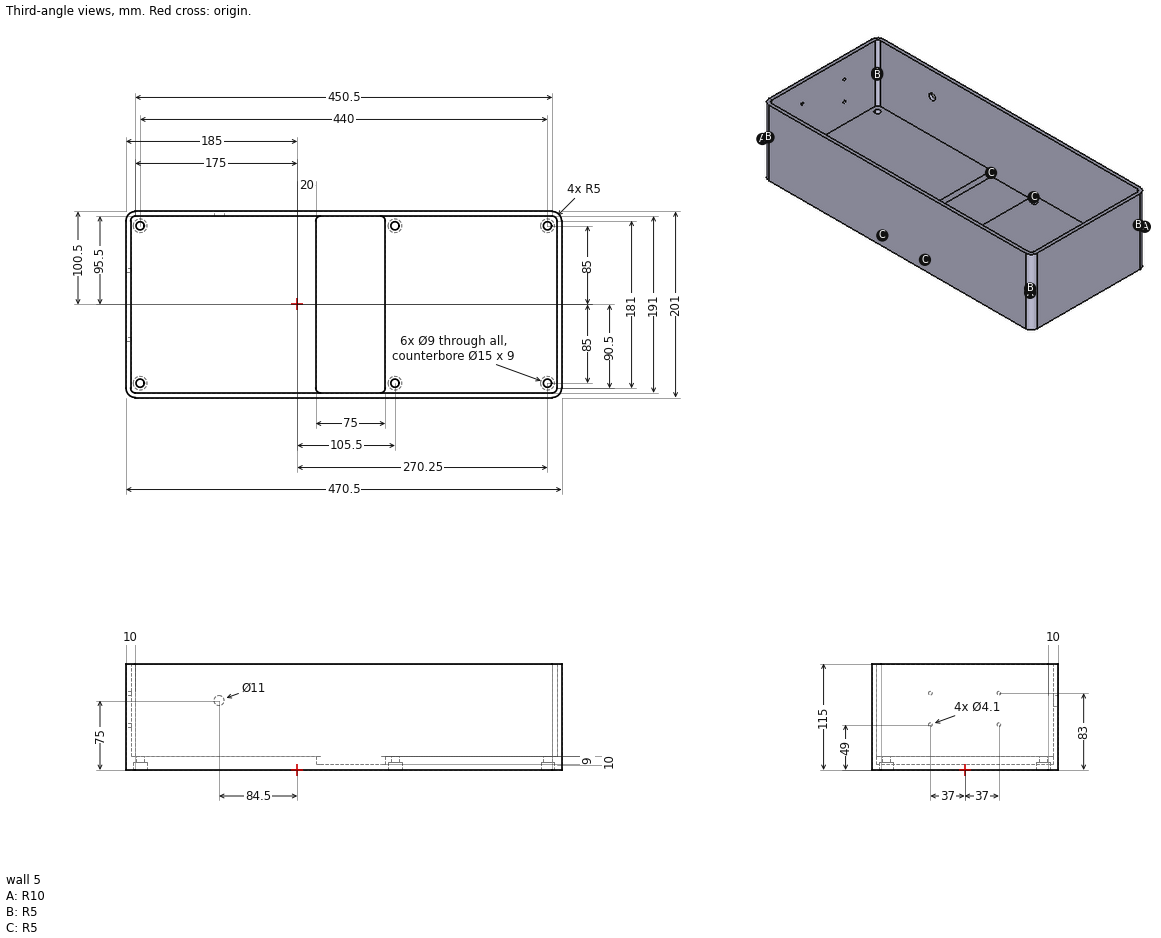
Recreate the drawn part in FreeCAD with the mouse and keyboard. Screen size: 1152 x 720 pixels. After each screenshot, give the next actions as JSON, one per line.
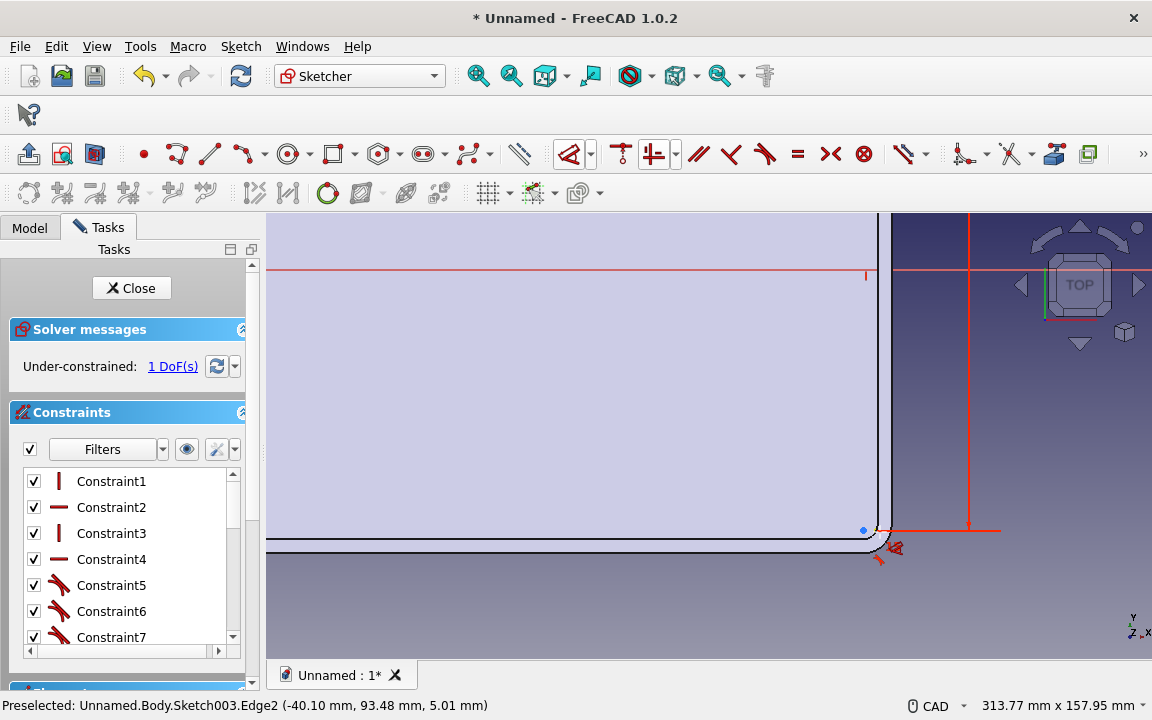
{"action": "left_click", "coordinate": [878, 531]}
{"action": "left_click", "coordinate": [912, 400]}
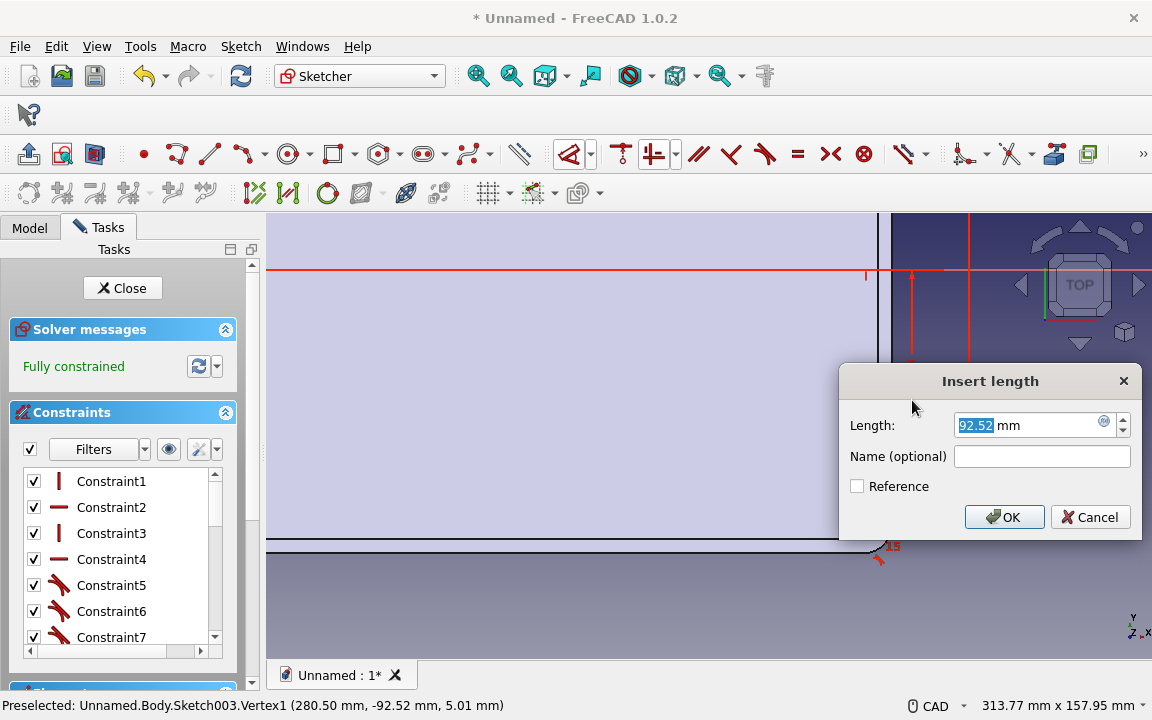
{"action": "type", "text": "90.5"}
{"action": "key", "text": "Return"}
{"action": "key", "text": "Escape"}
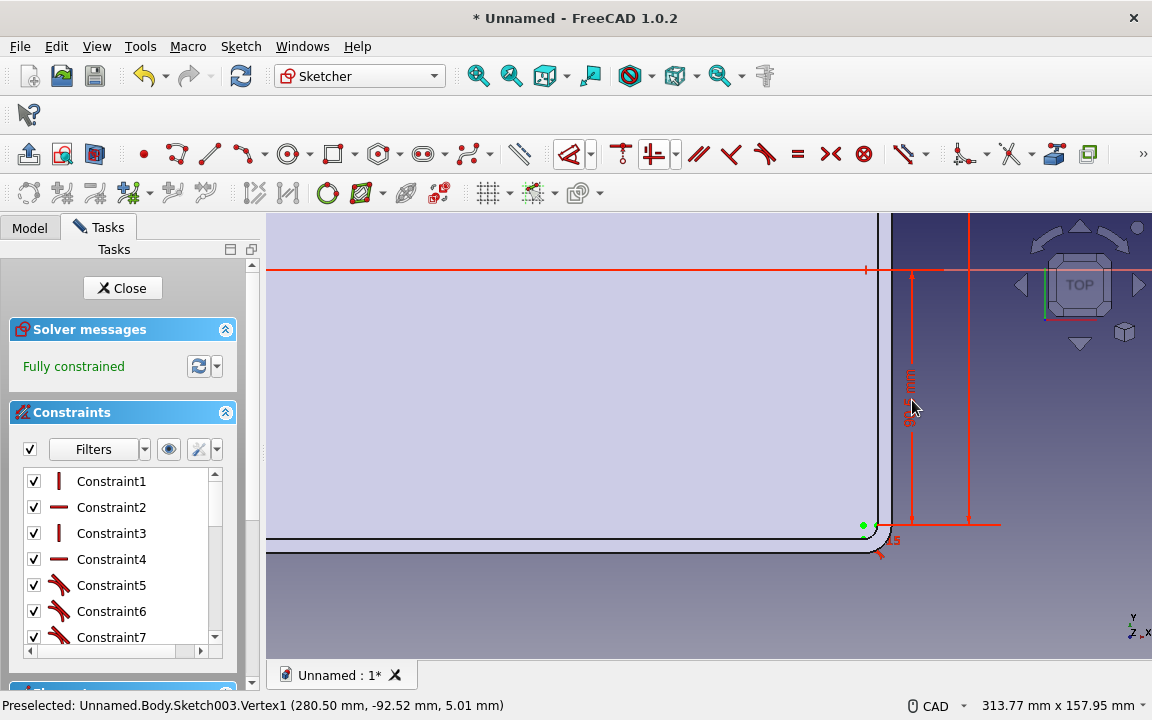
{"action": "left_click", "coordinate": [123, 288]}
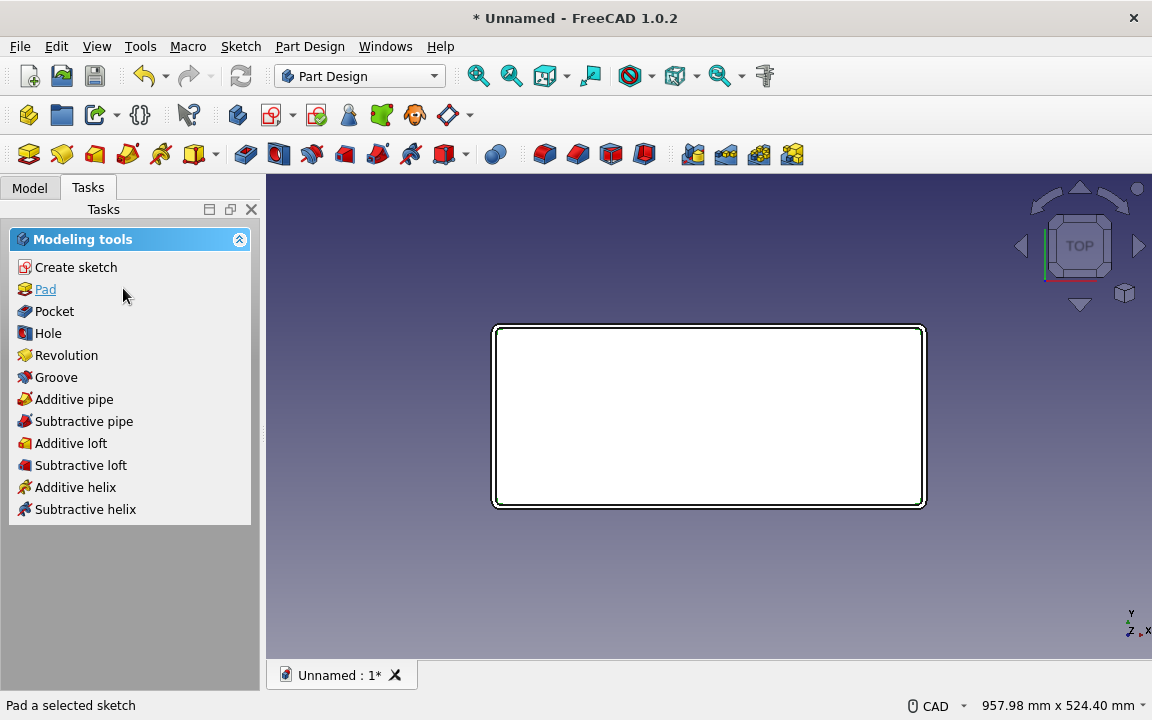
{"action": "left_click", "coordinate": [29, 154]}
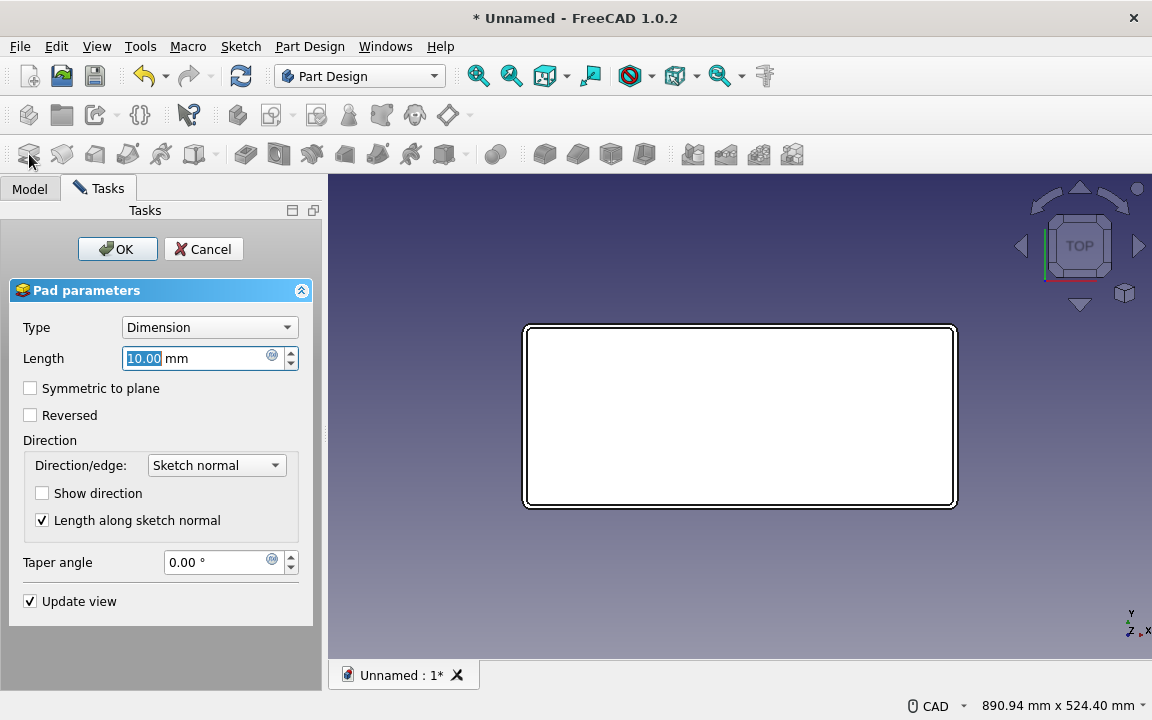
{"action": "type", "text": "10"}
{"action": "key", "text": "Tab"}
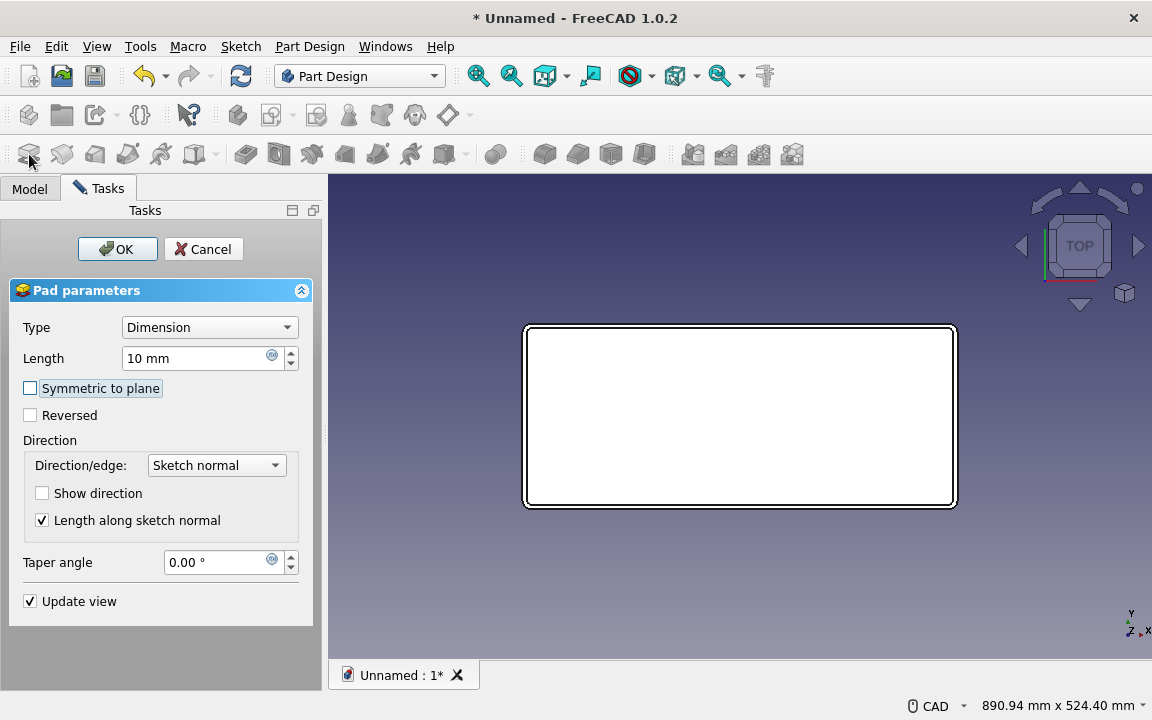
{"action": "left_click", "coordinate": [118, 249]}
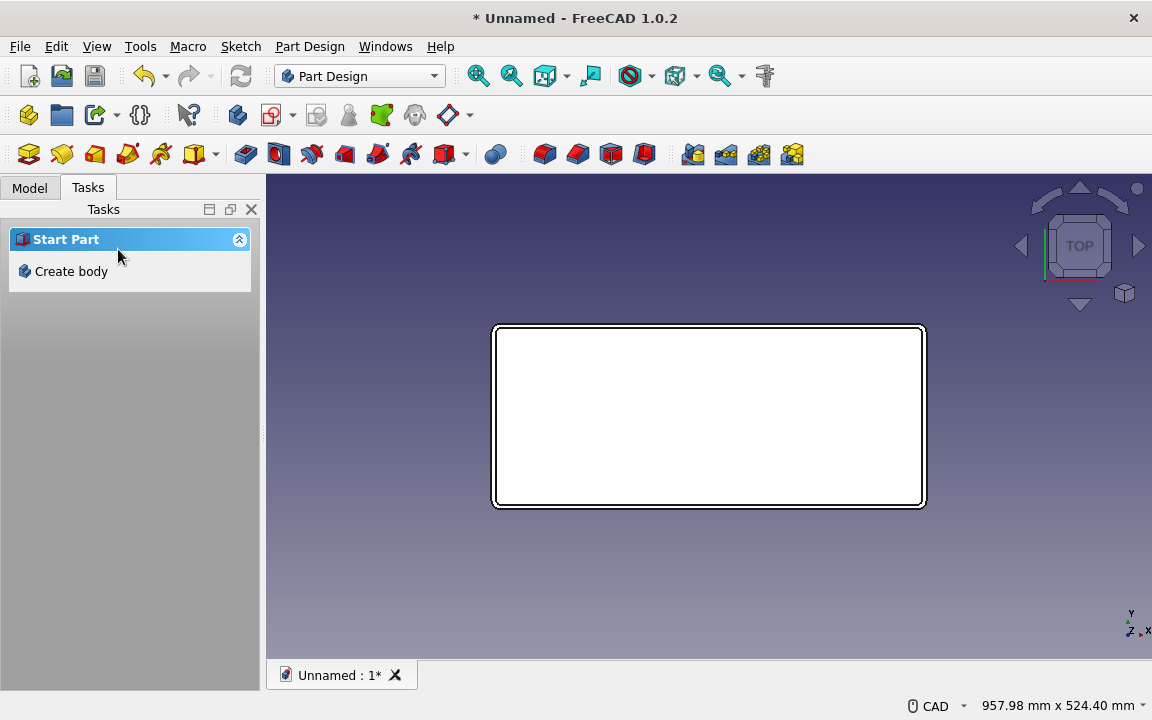
{"action": "key", "text": "5"}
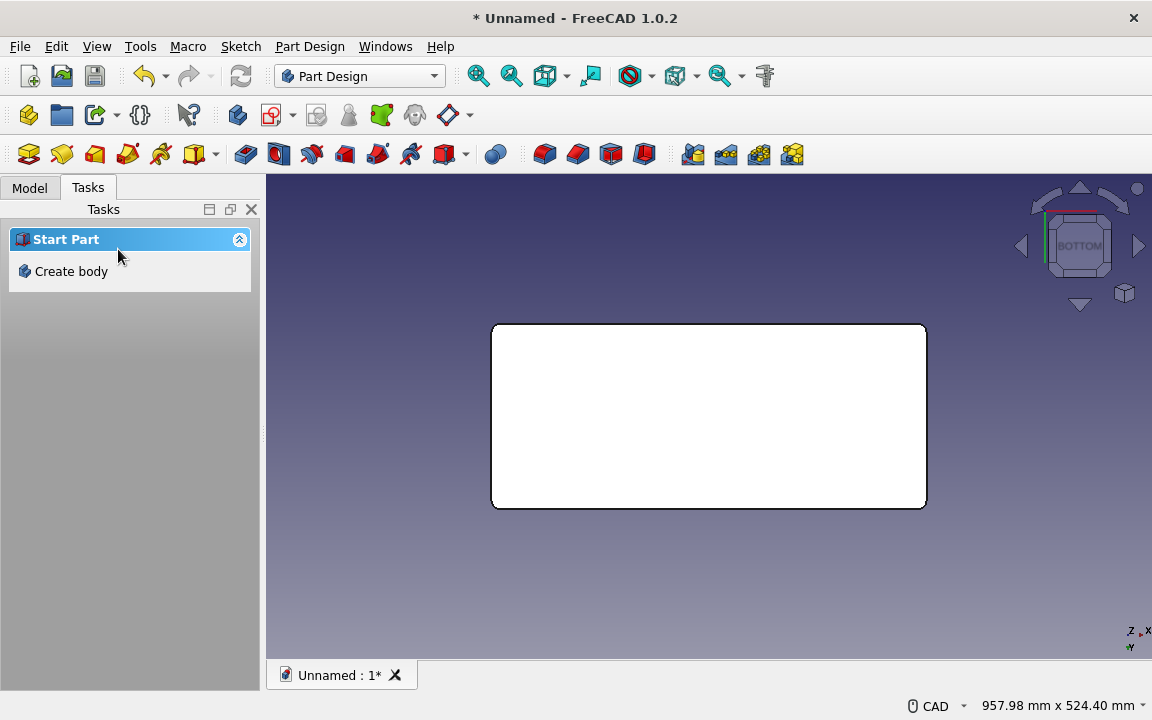
{"action": "left_click", "coordinate": [833, 415]}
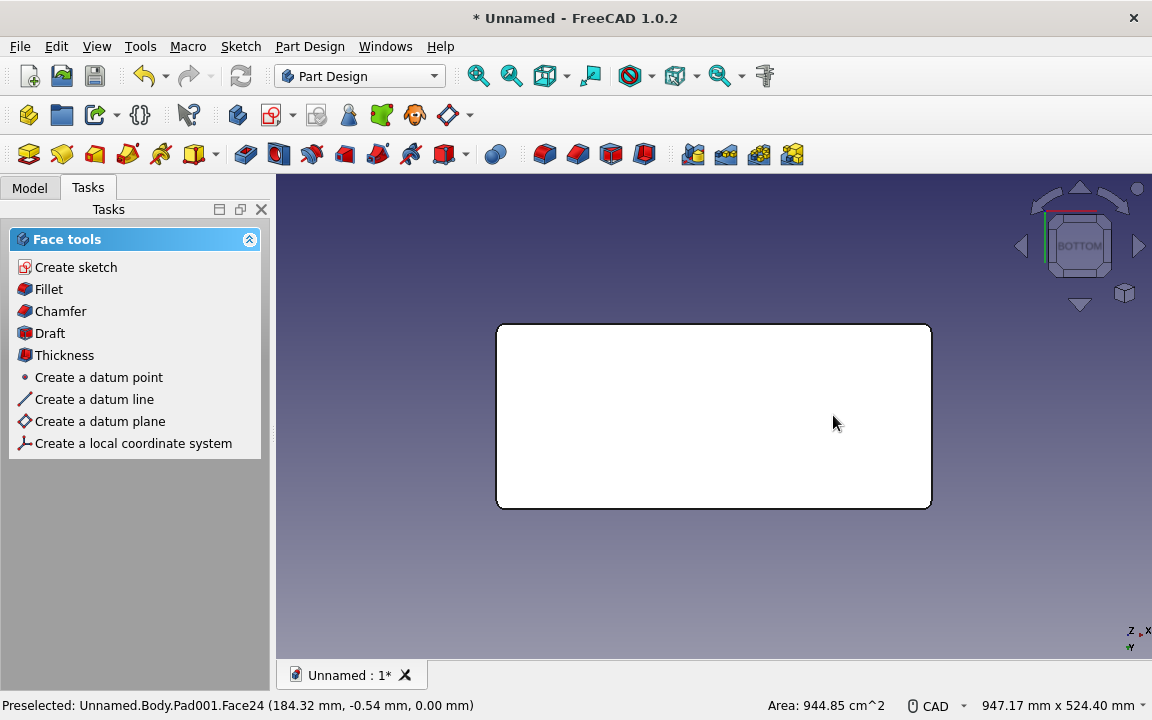
{"action": "left_click", "coordinate": [270, 116]}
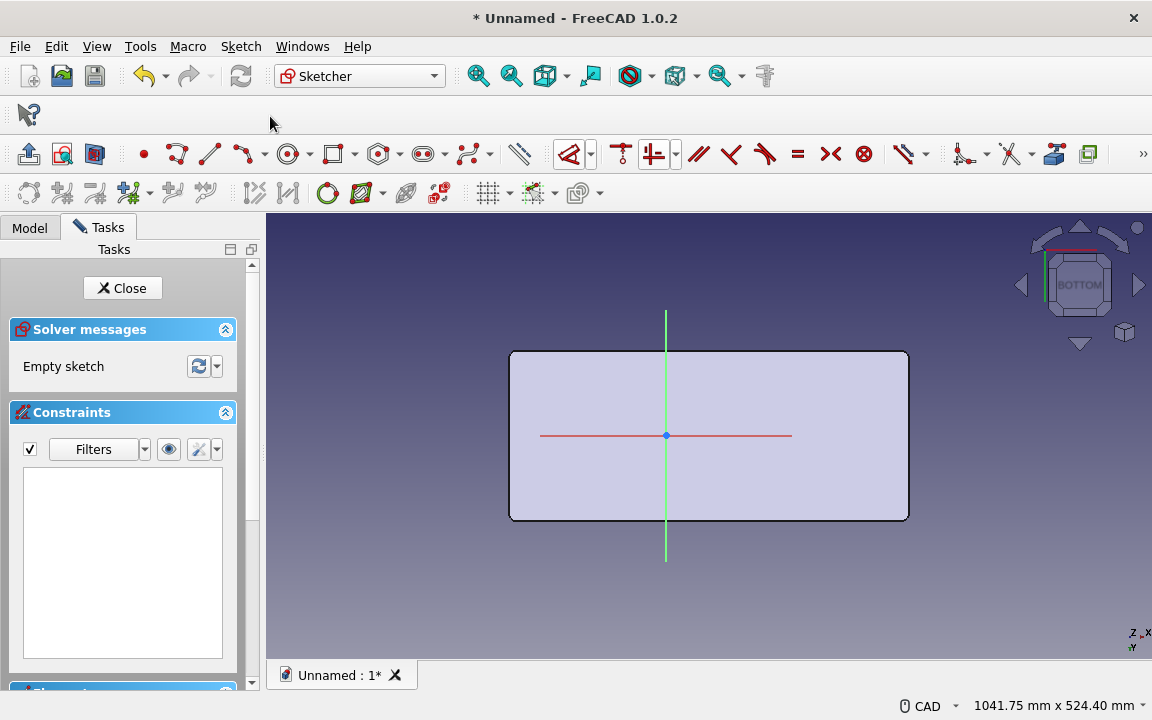
{"action": "key", "text": "g c"}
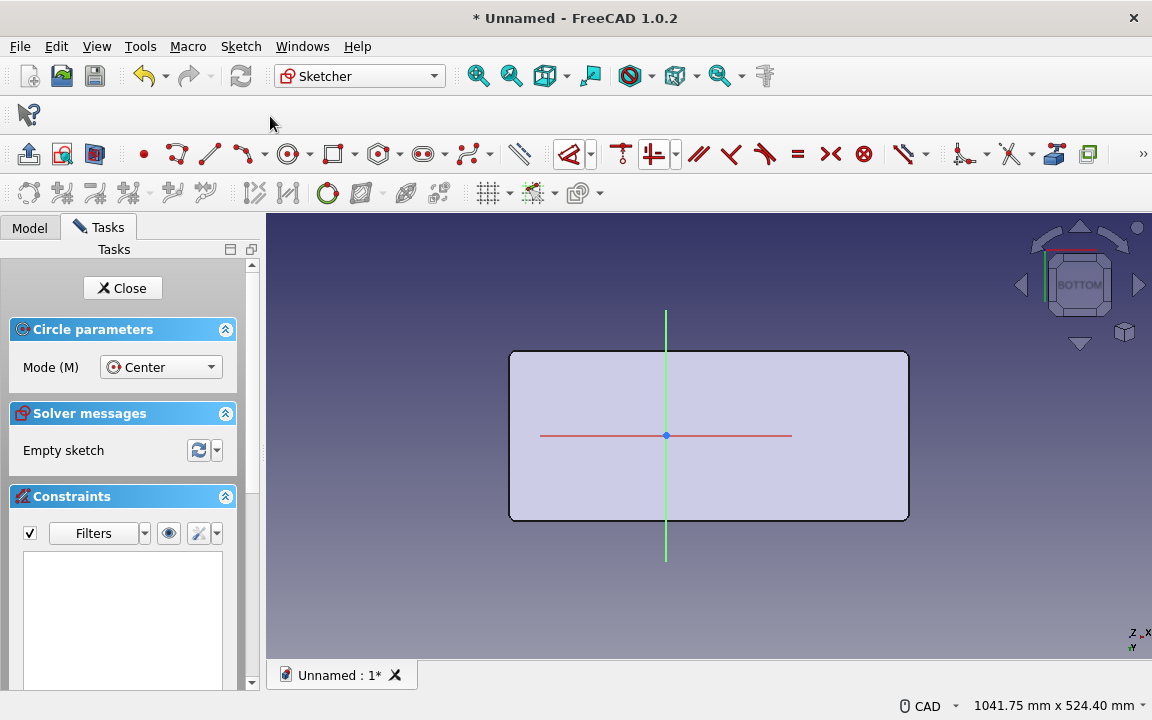
{"action": "scroll", "coordinate": [896, 364], "scroll_direction": "up", "scroll_amount": 9}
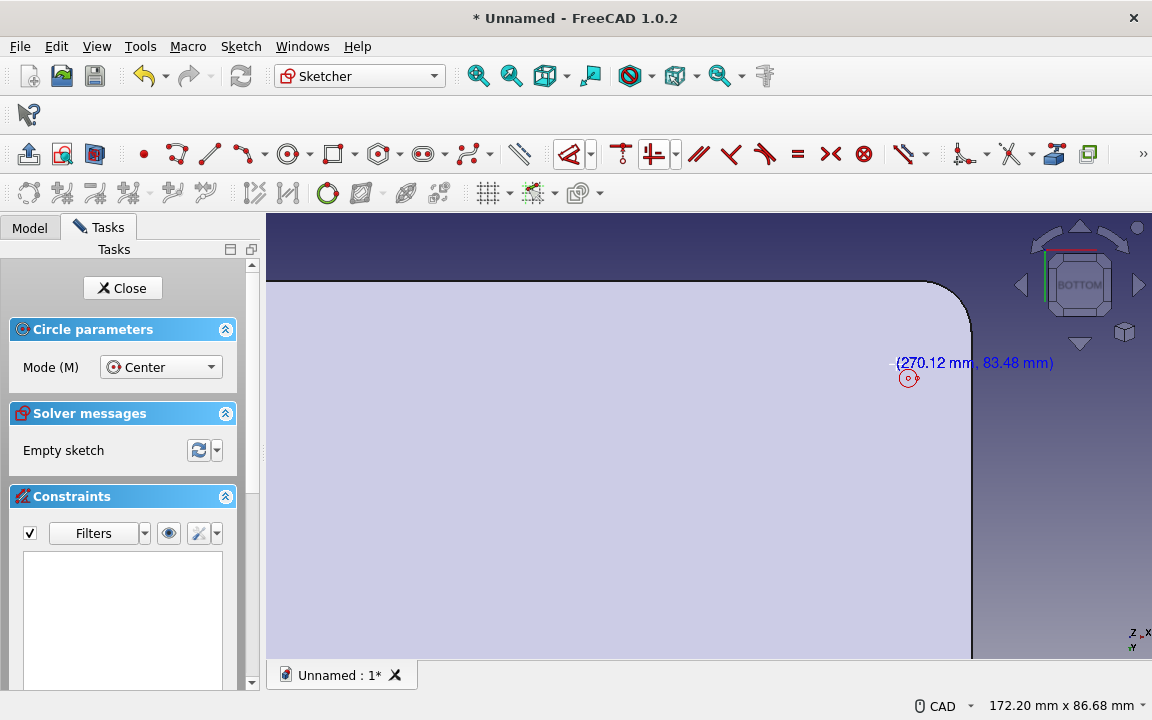
{"action": "scroll", "coordinate": [863, 344], "scroll_direction": "down", "scroll_amount": 8}